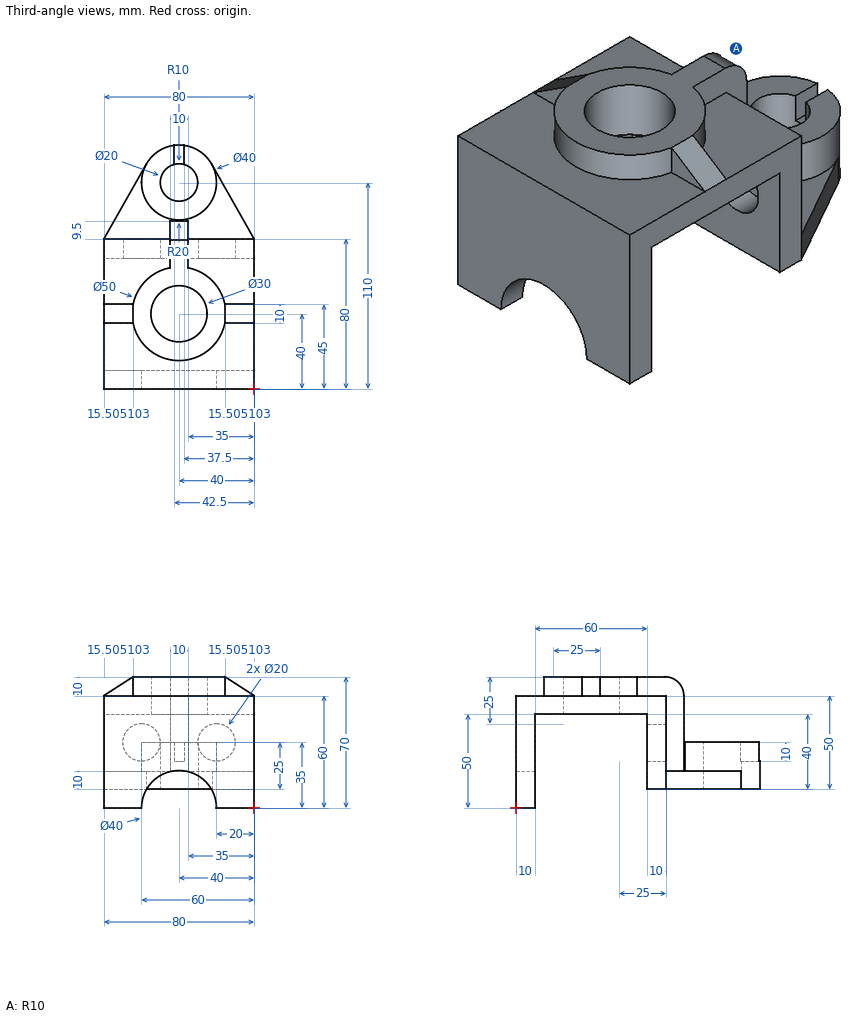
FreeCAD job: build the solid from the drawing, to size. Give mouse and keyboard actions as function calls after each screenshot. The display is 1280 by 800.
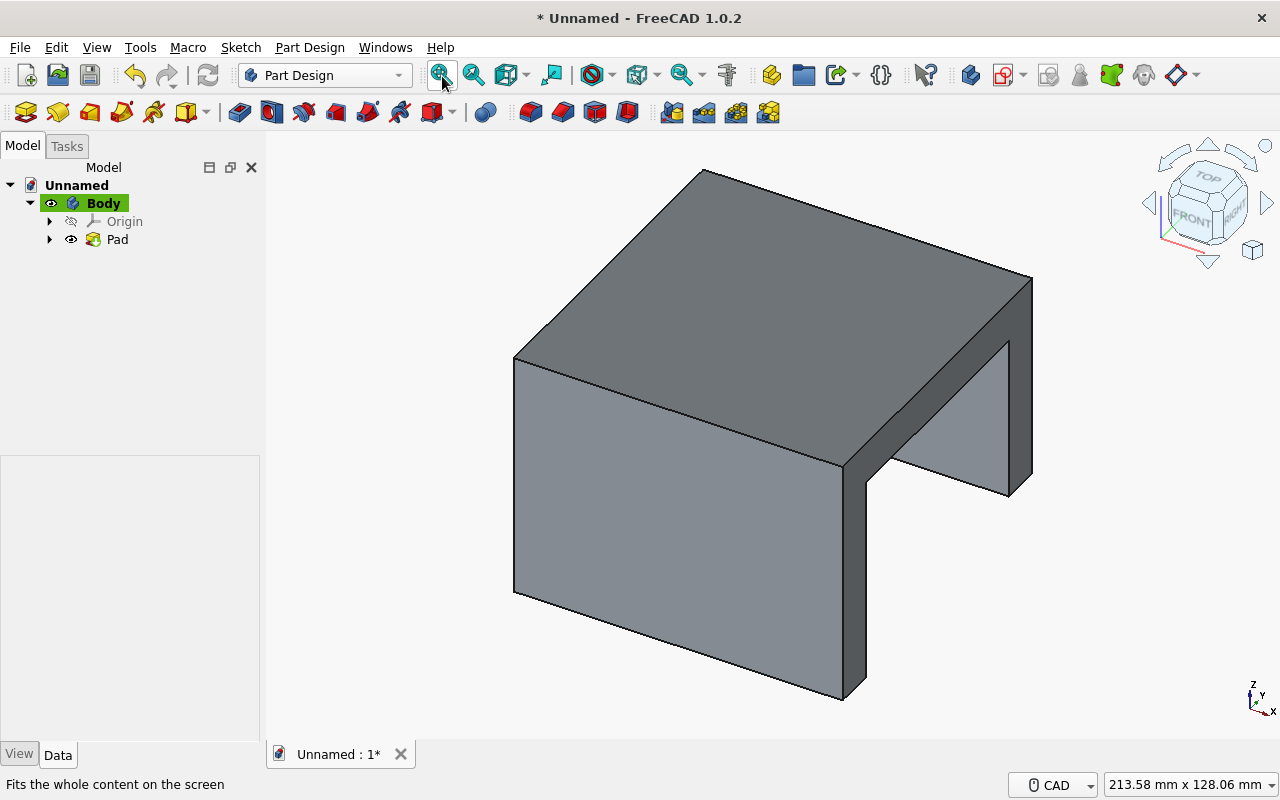
click(773, 317)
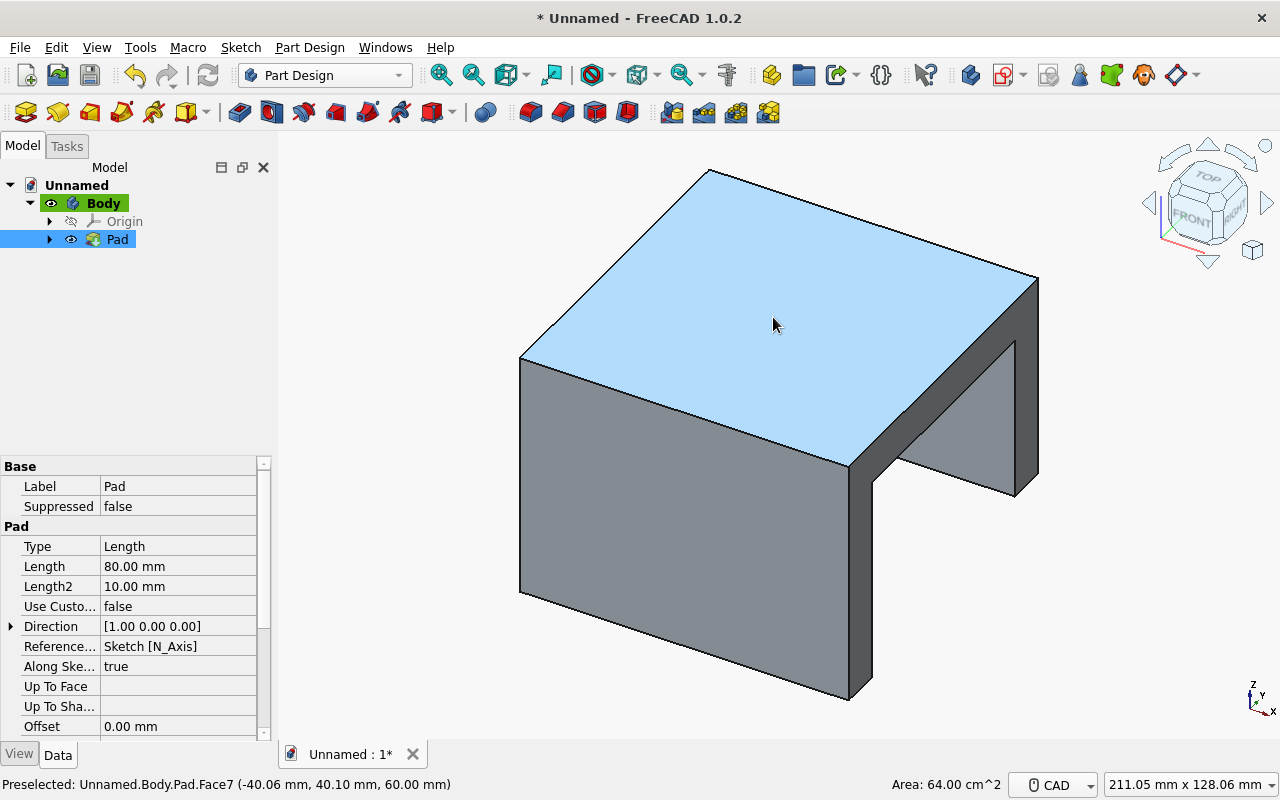
click(1004, 76)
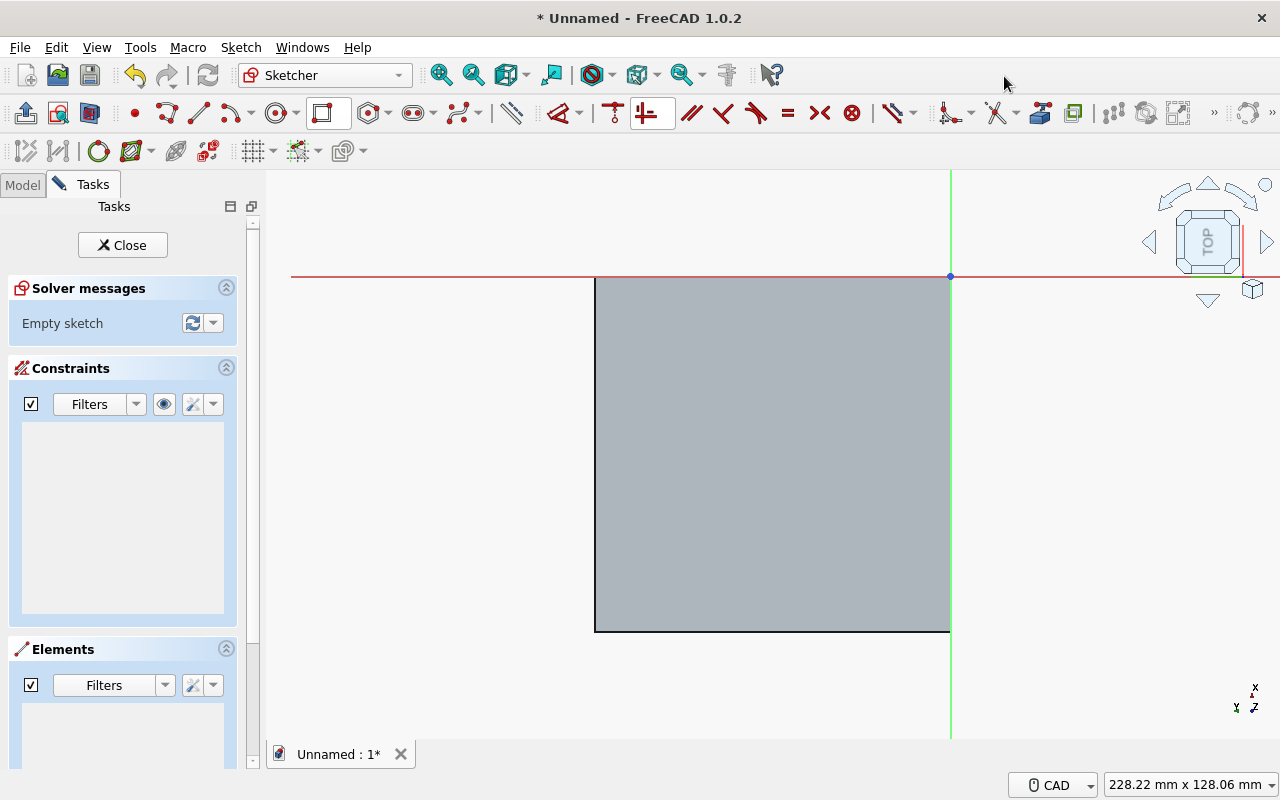
click(276, 114)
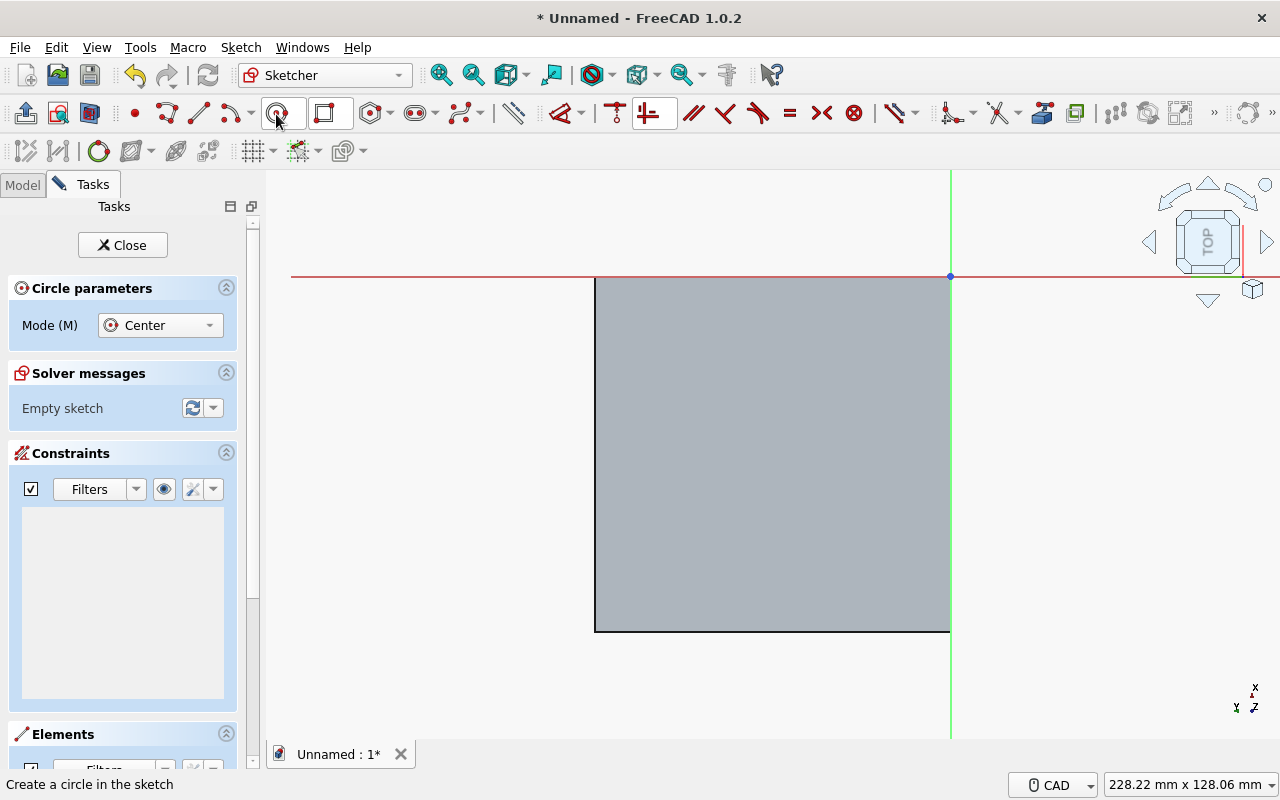
click(773, 455)
move(852, 376)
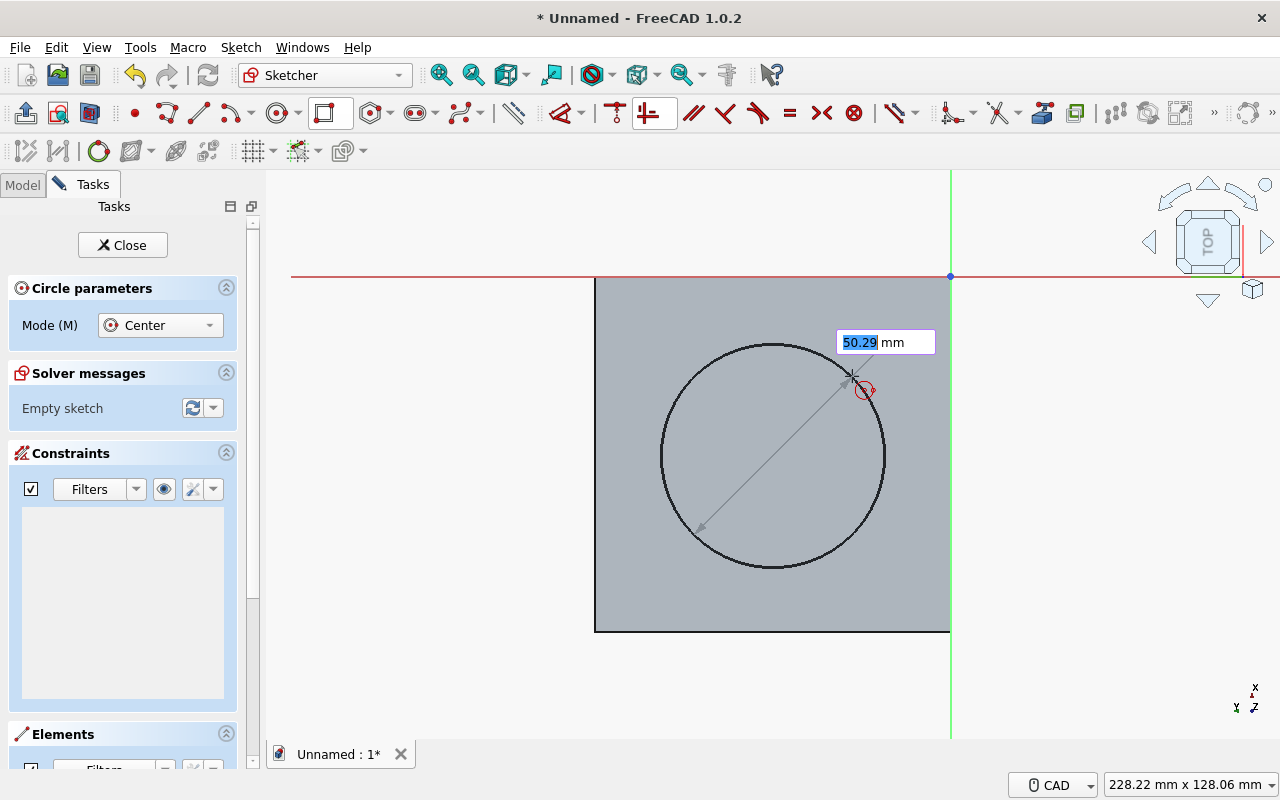
text(50)
key(Return)
key(Escape)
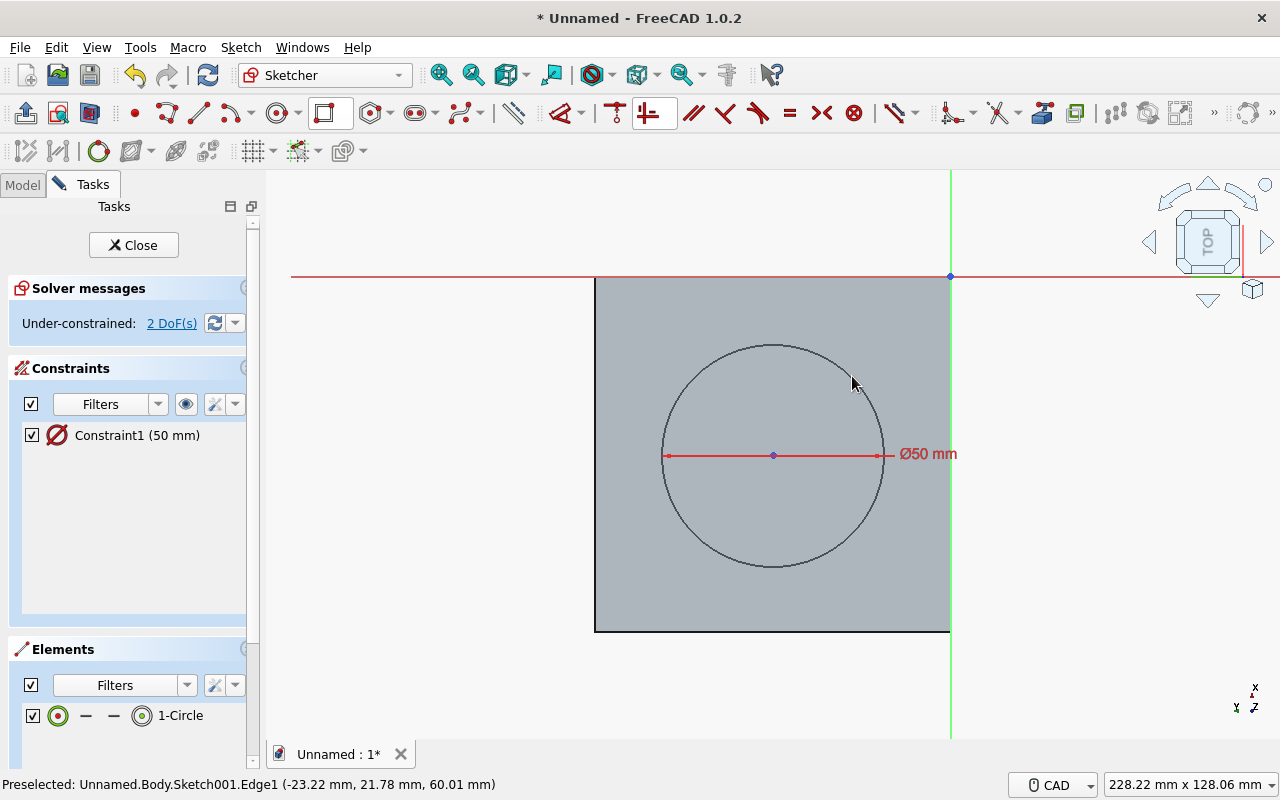
click(560, 114)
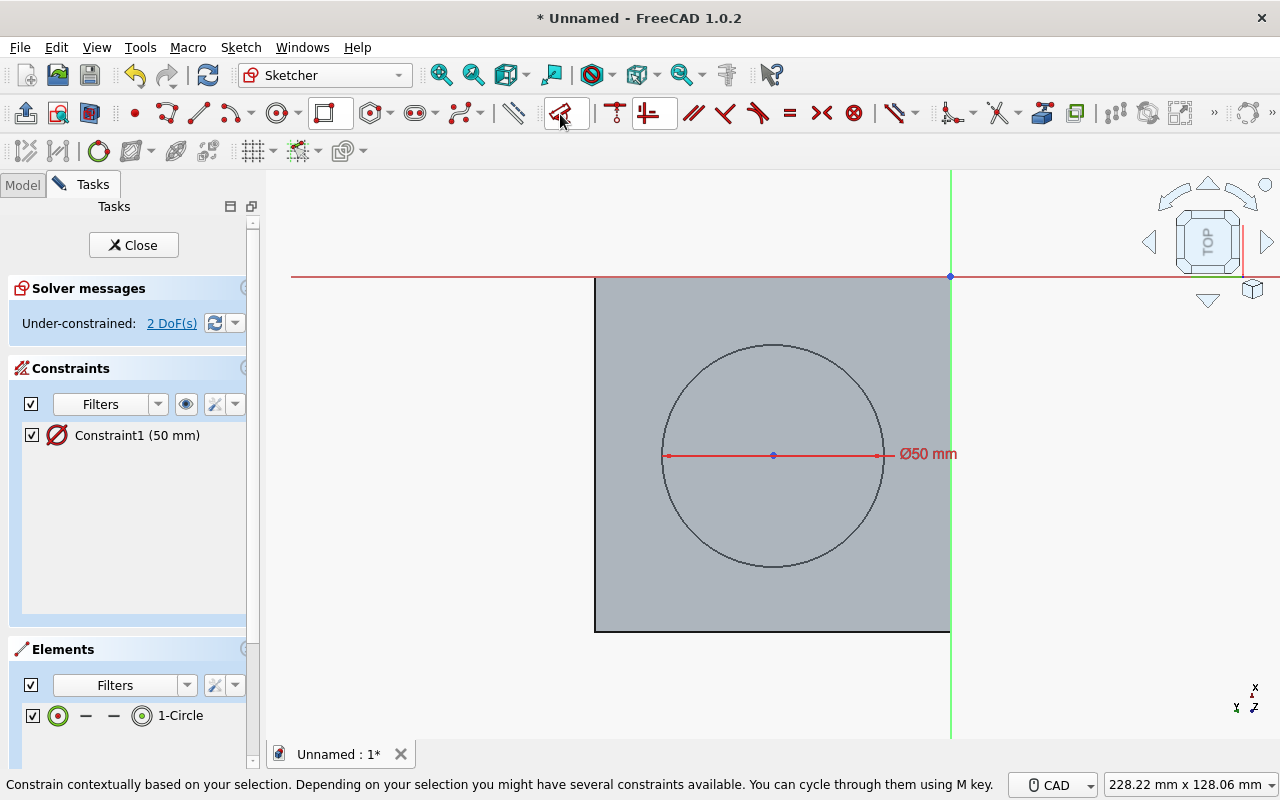
click(773, 456)
click(862, 243)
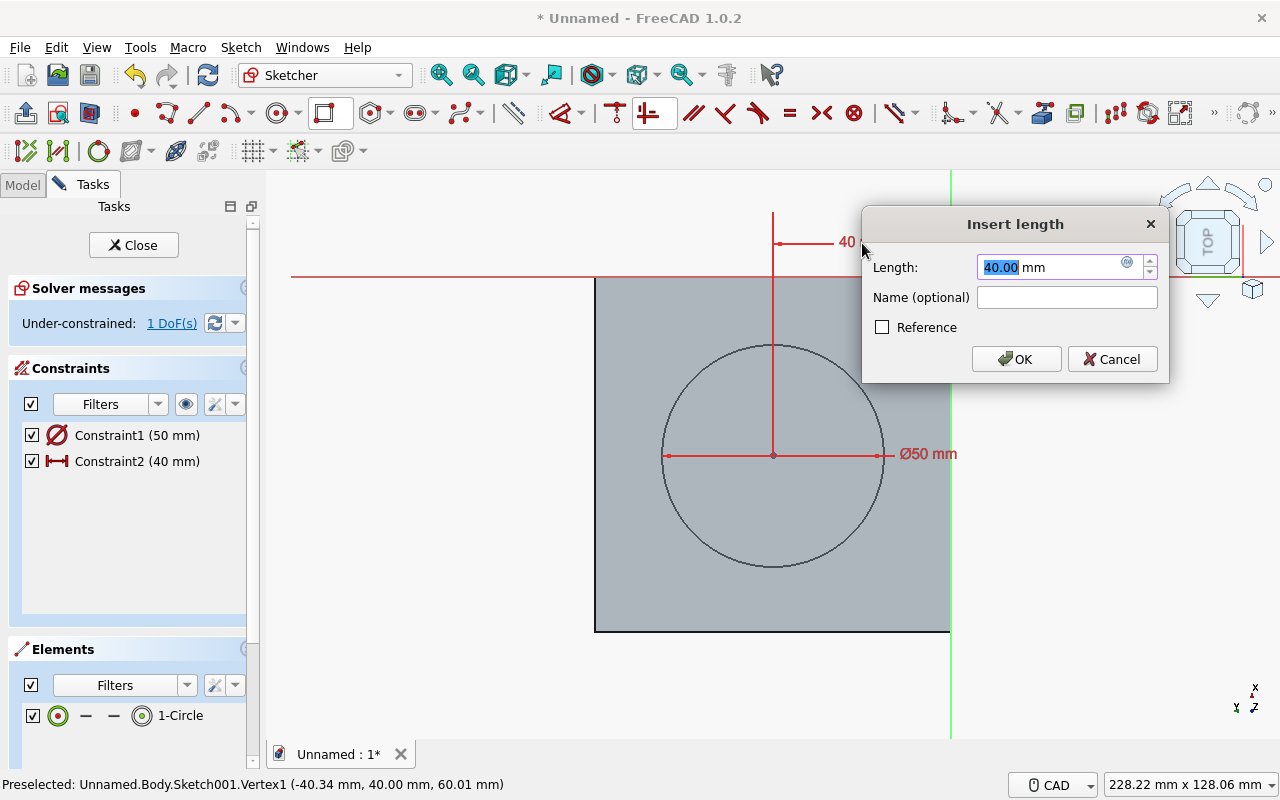
text(40)
key(Return)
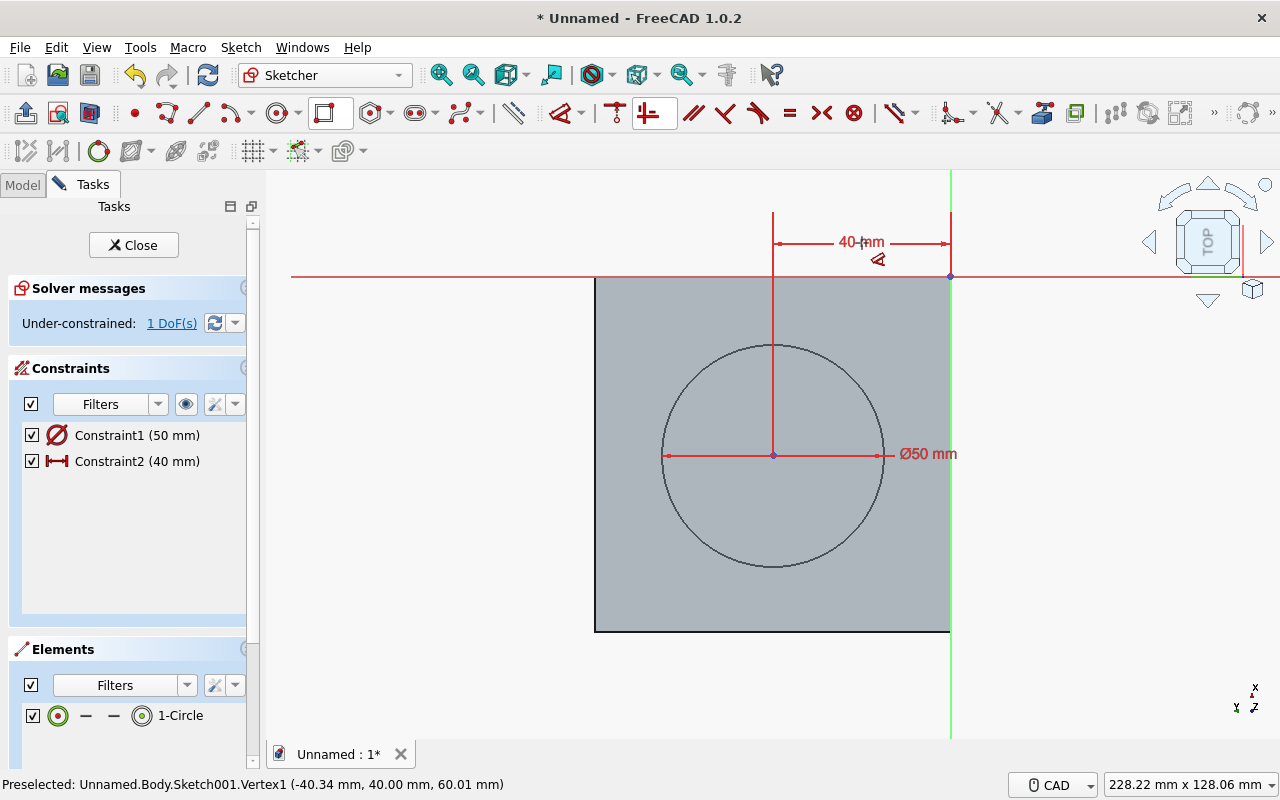
click(773, 456)
click(985, 366)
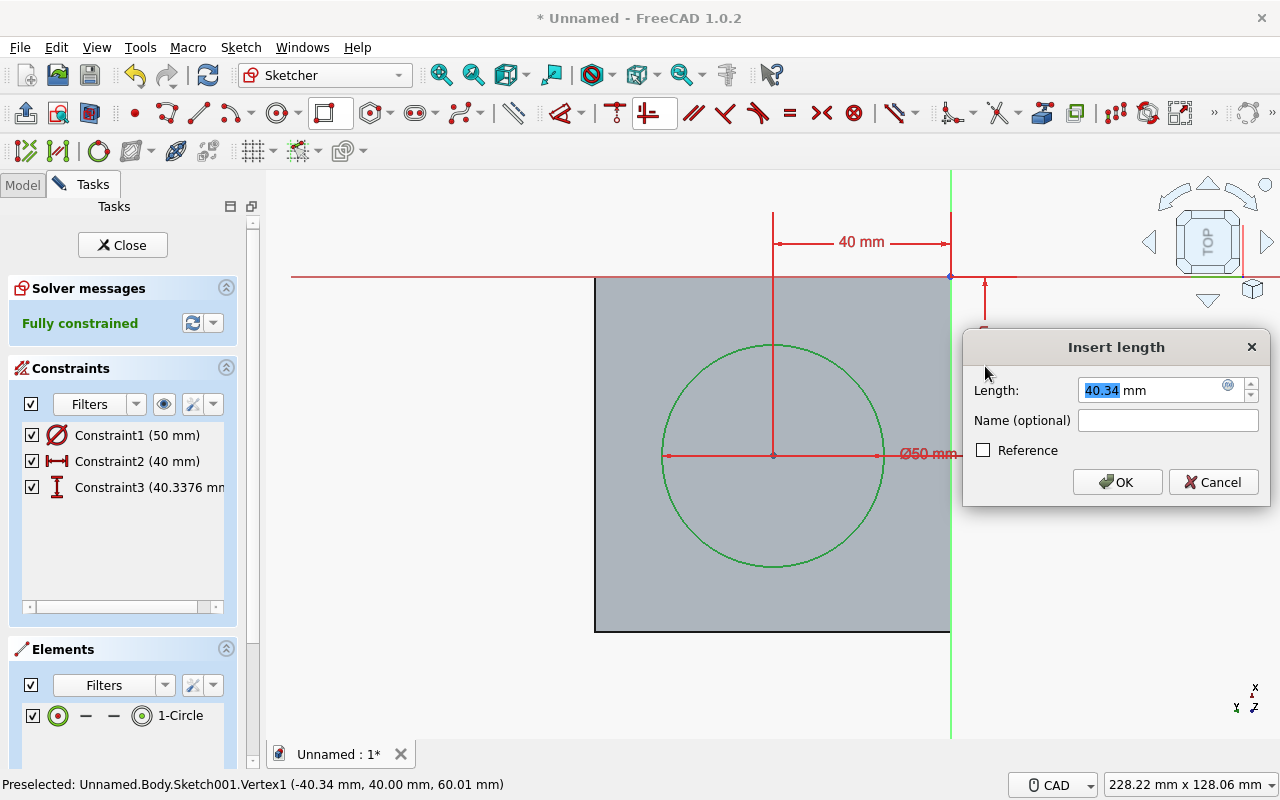
text(40)
key(Return)
key(Escape)